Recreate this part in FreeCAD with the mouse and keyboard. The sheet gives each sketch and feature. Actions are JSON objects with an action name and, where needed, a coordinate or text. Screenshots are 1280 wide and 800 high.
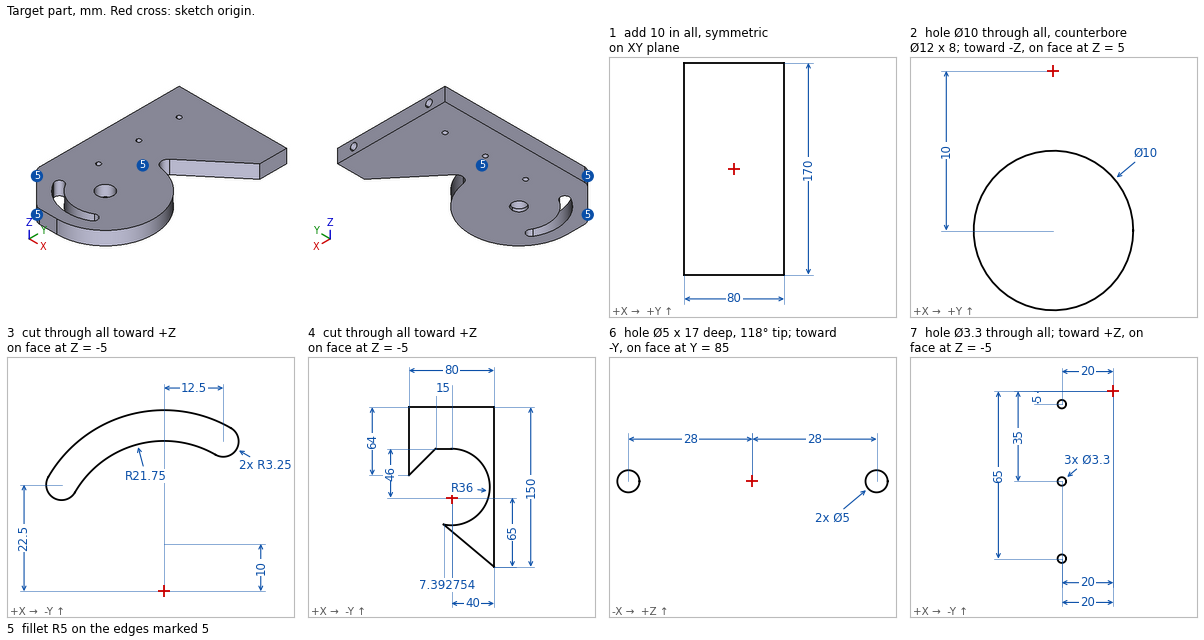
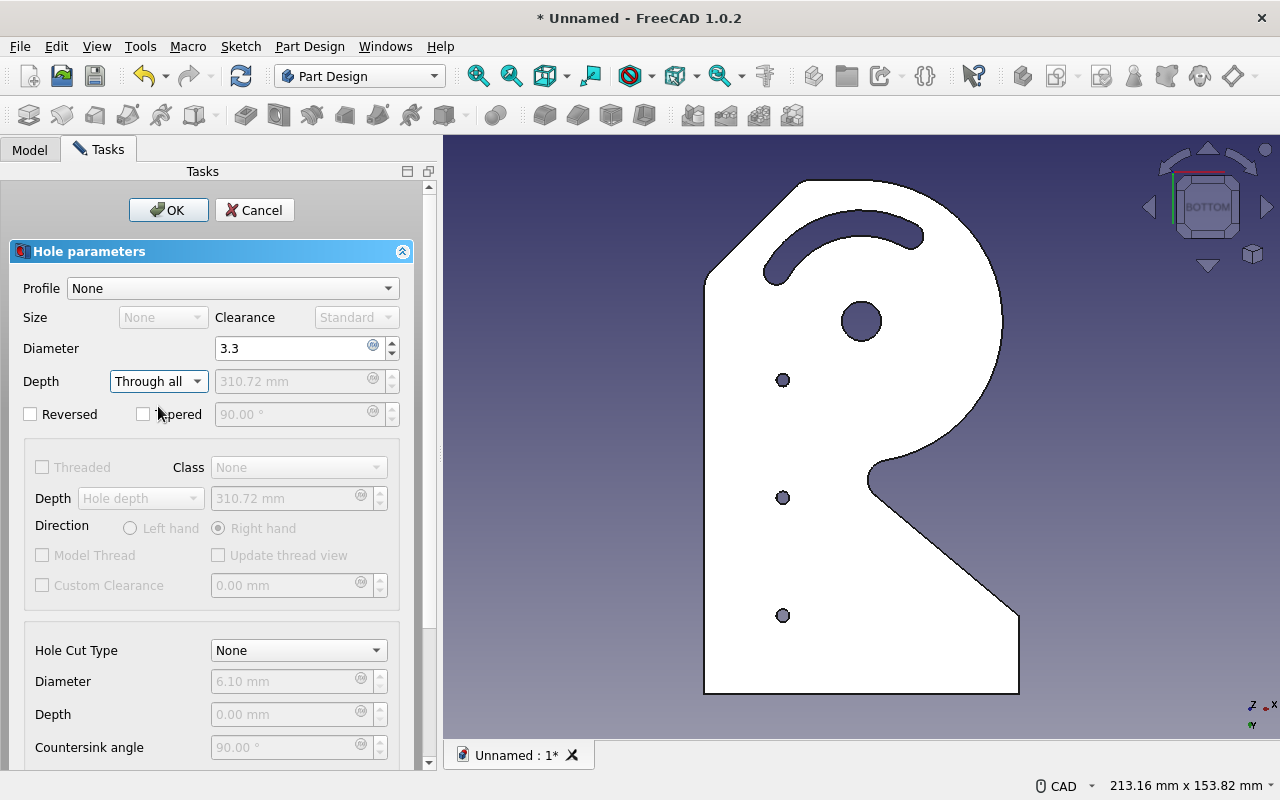
{"action": "left_click", "coordinate": [169, 210]}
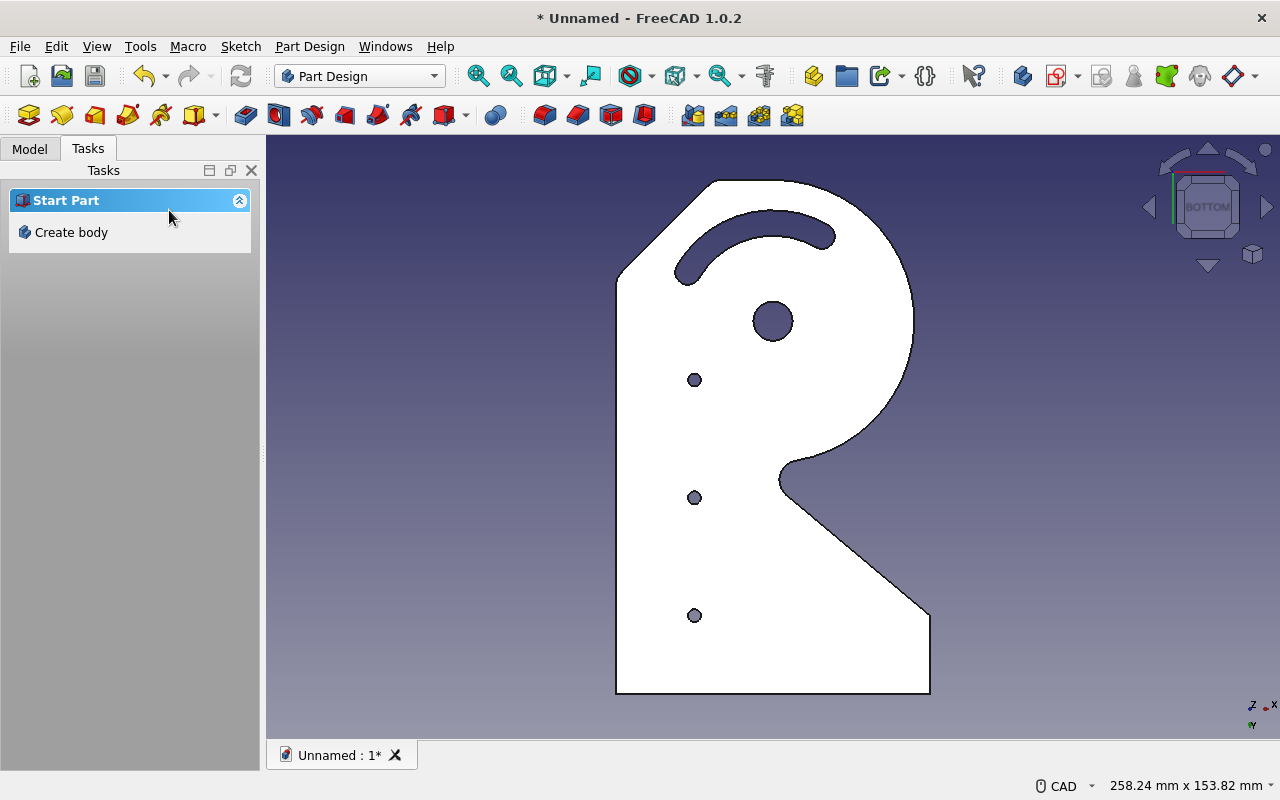
{"action": "key", "text": "0"}